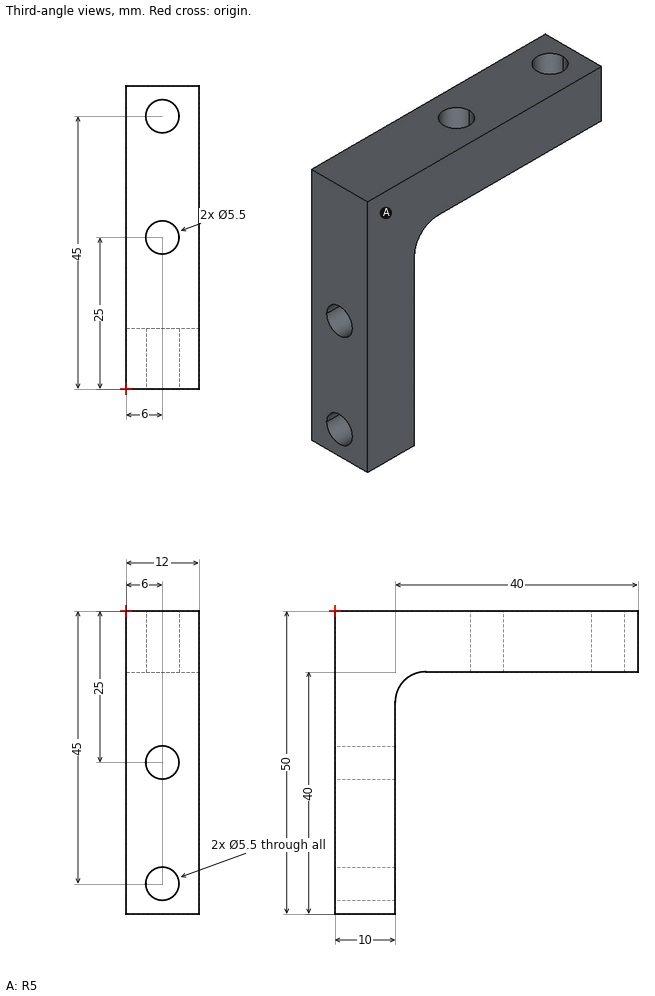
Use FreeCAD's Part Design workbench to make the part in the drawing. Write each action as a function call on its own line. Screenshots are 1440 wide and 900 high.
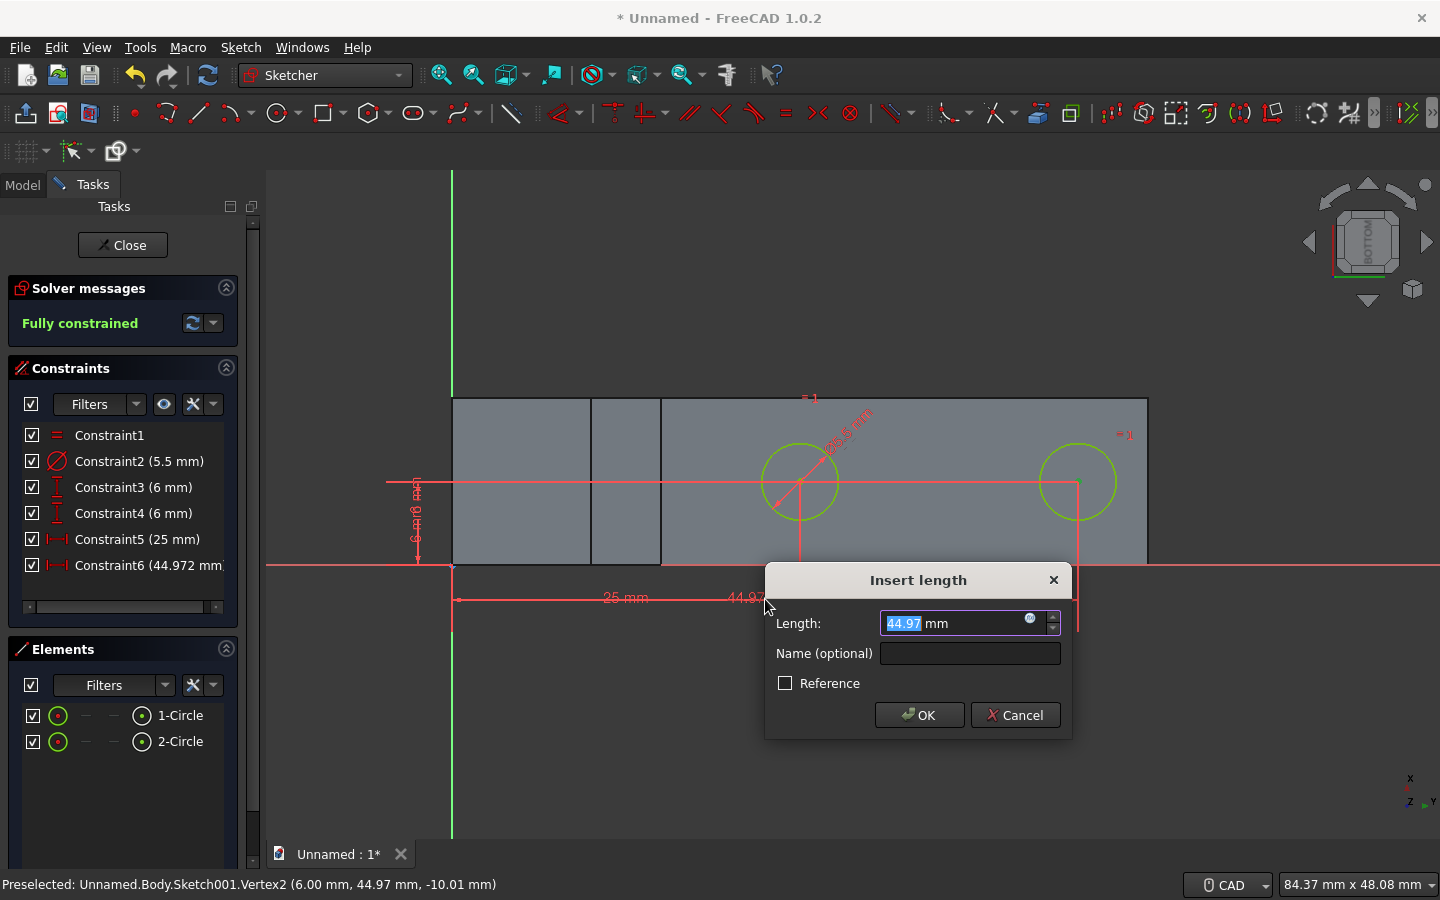
text(45)
key(Return)
key(Escape)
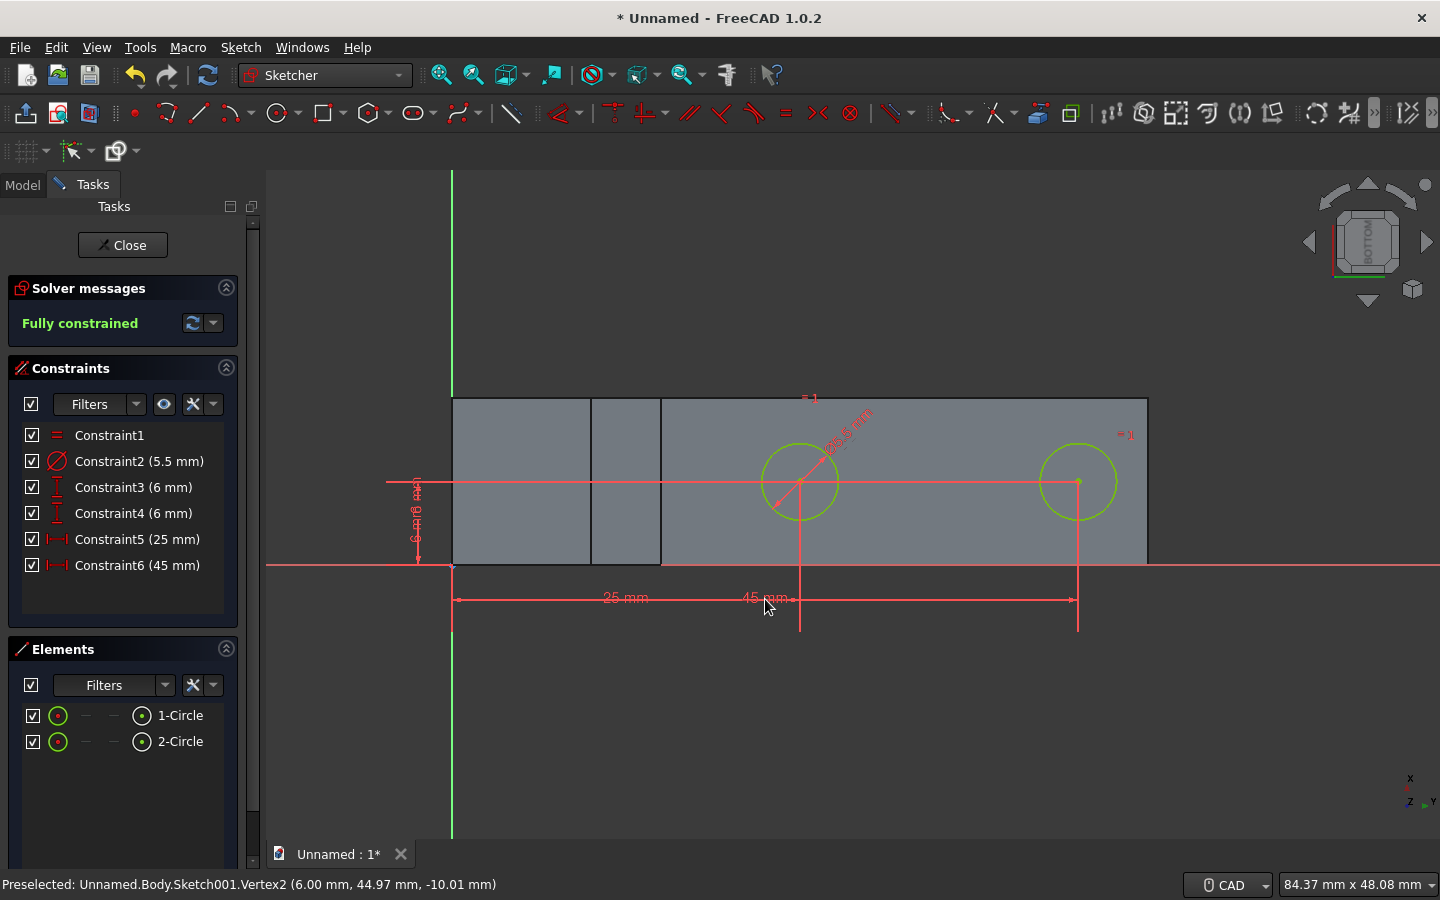
click(123, 245)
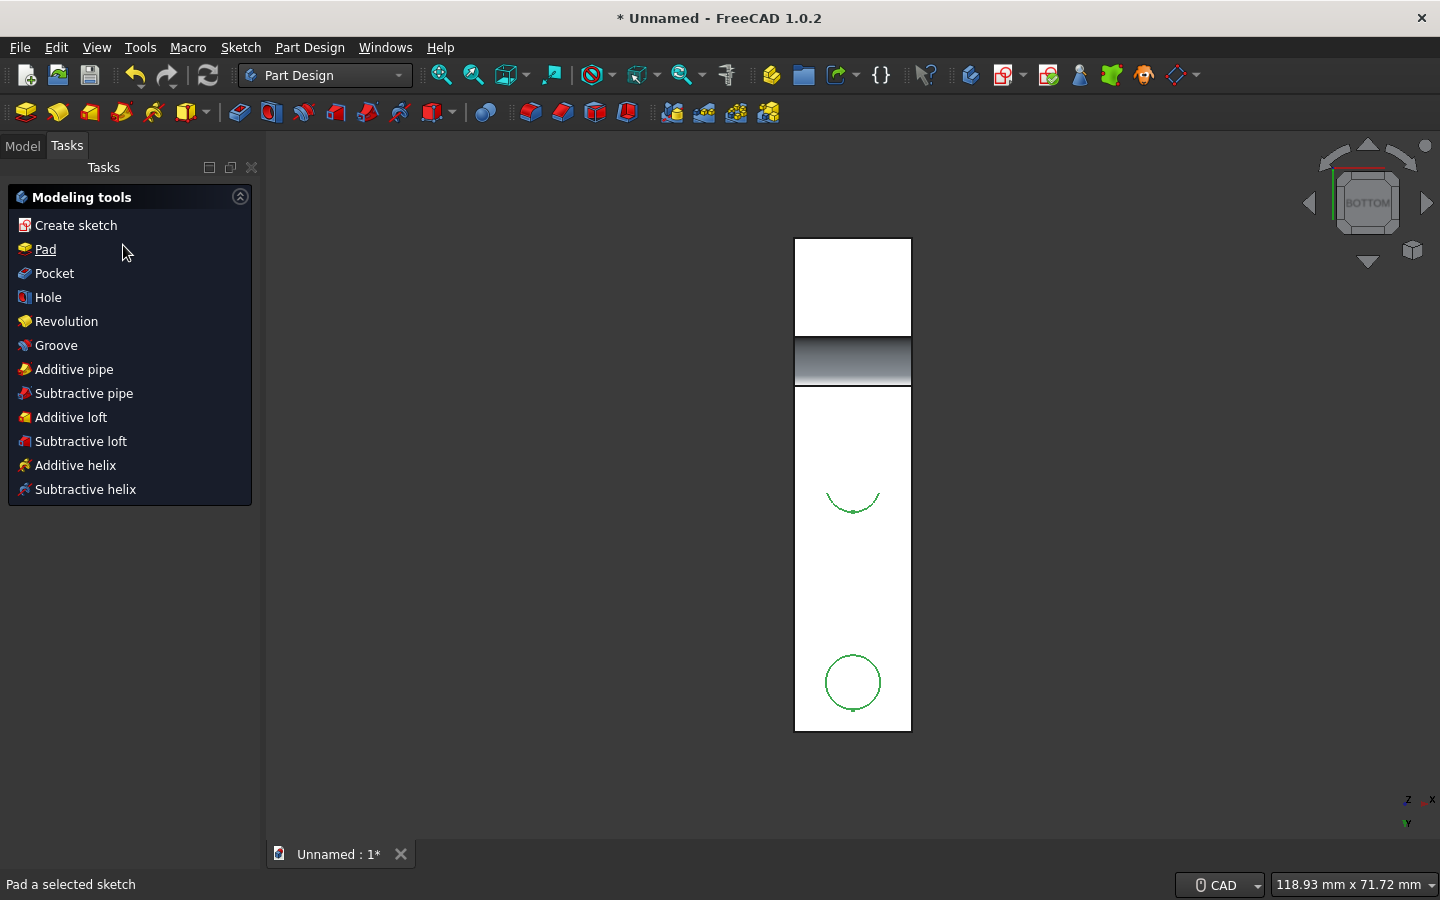
click(240, 112)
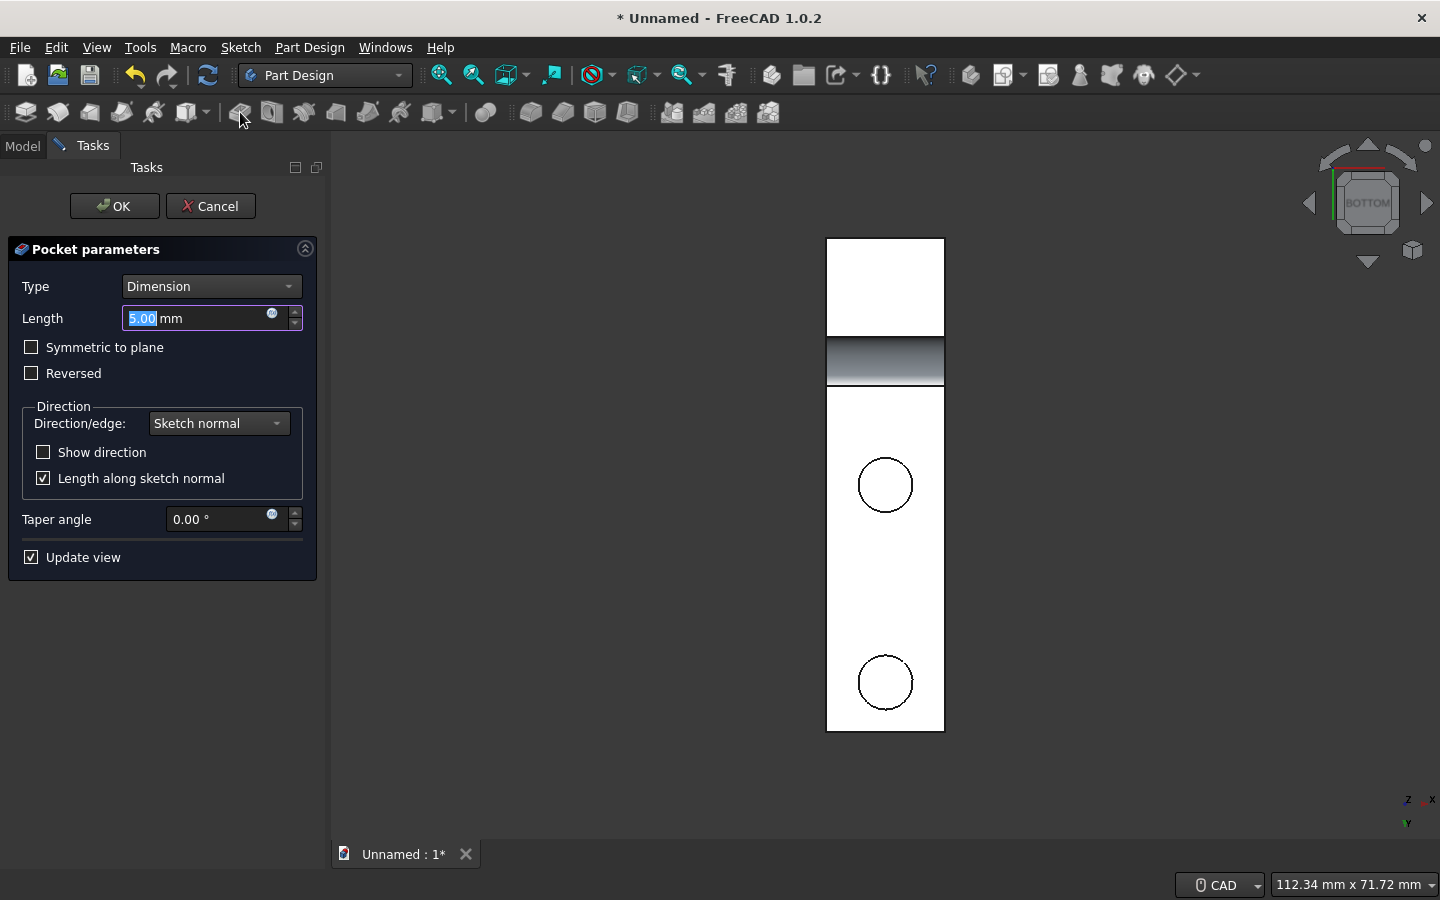
click(212, 286)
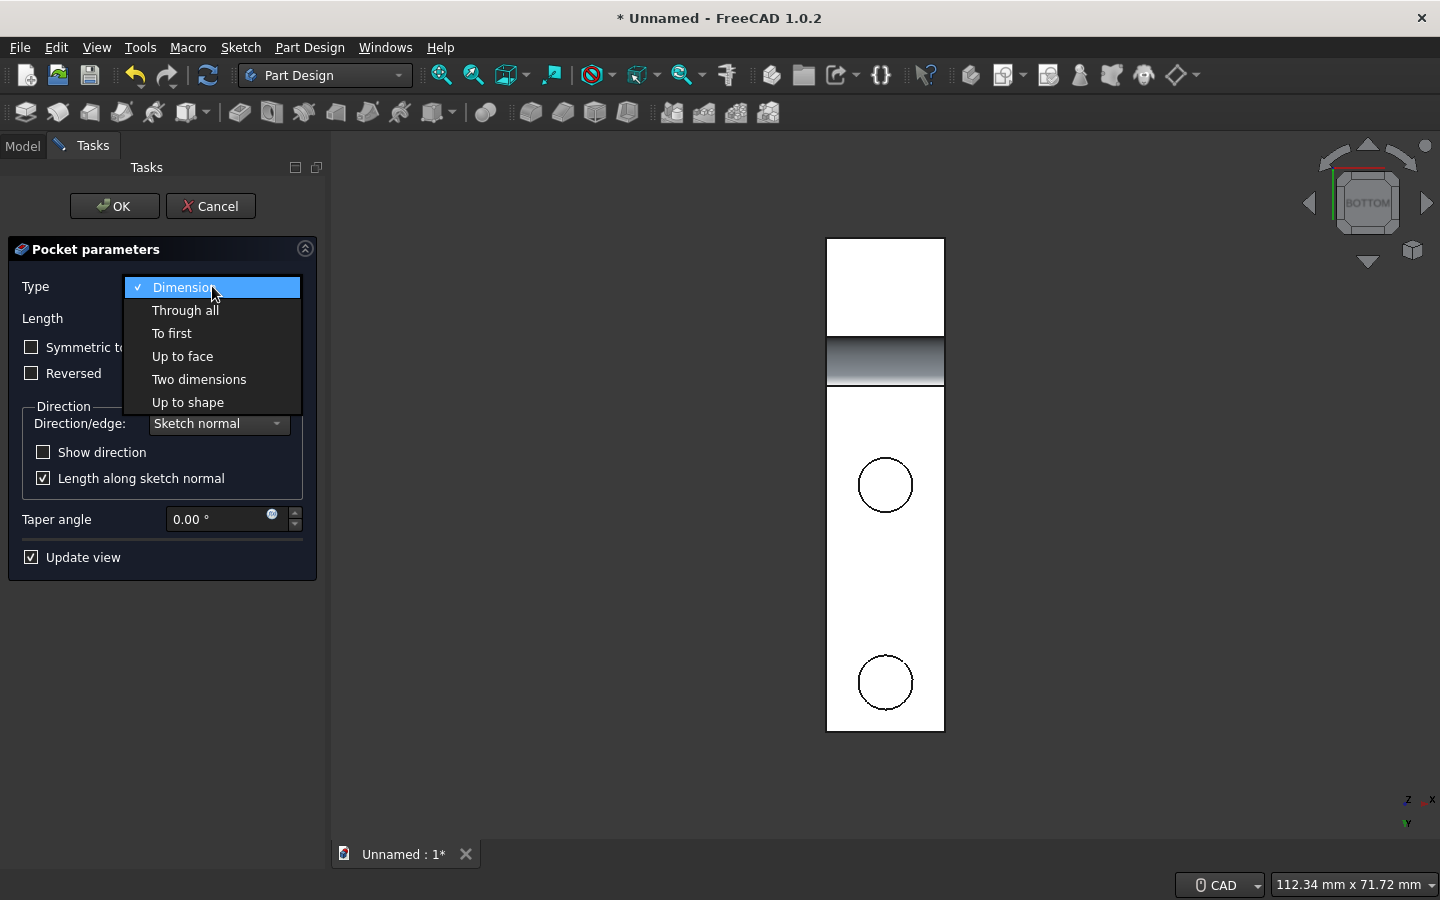
click(212, 310)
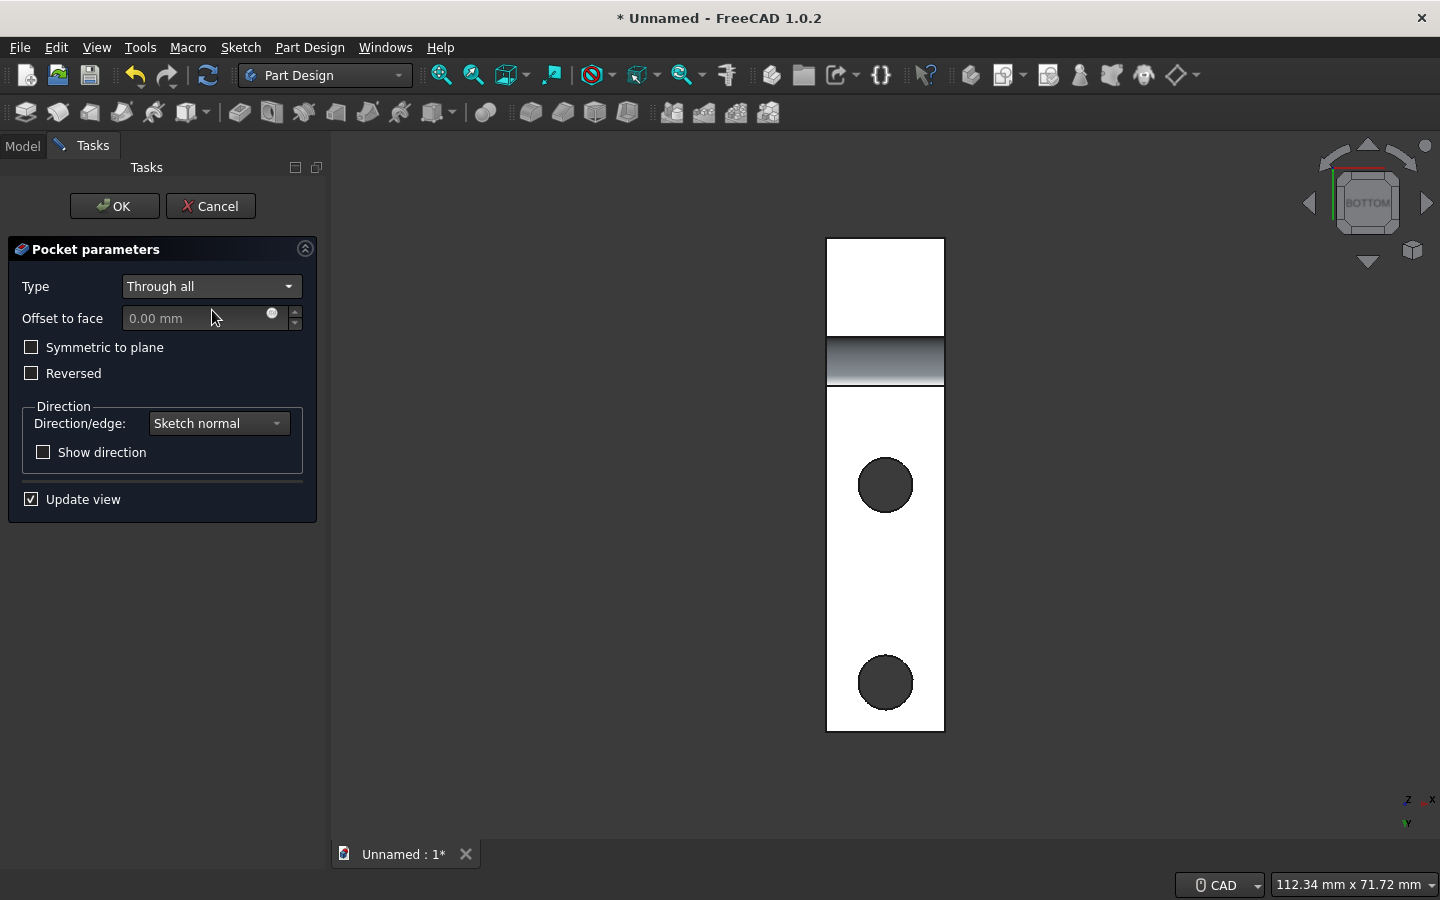
click(115, 206)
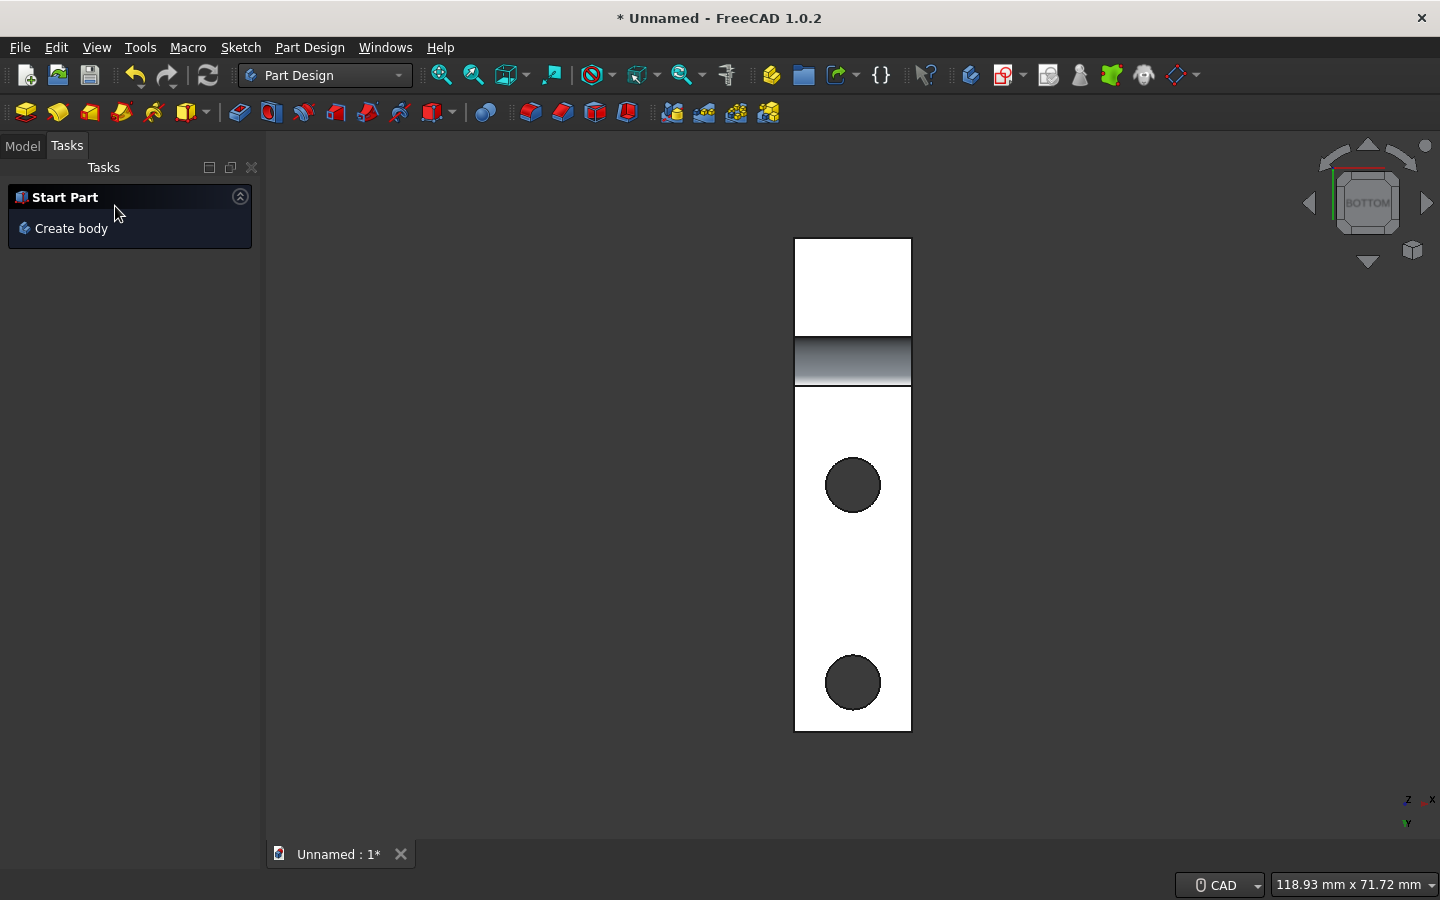
key(4)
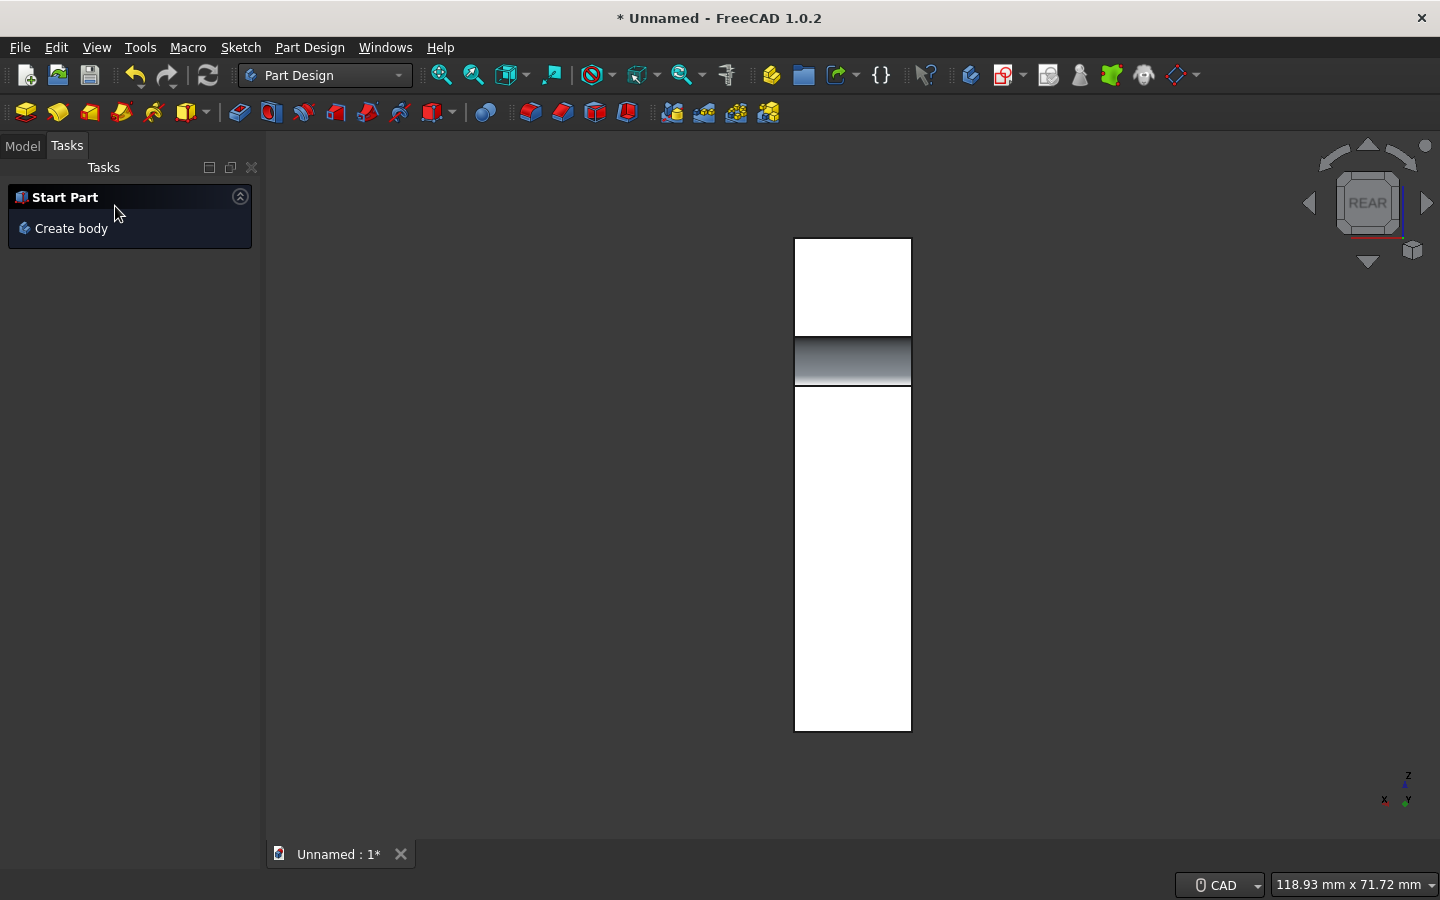
click(853, 558)